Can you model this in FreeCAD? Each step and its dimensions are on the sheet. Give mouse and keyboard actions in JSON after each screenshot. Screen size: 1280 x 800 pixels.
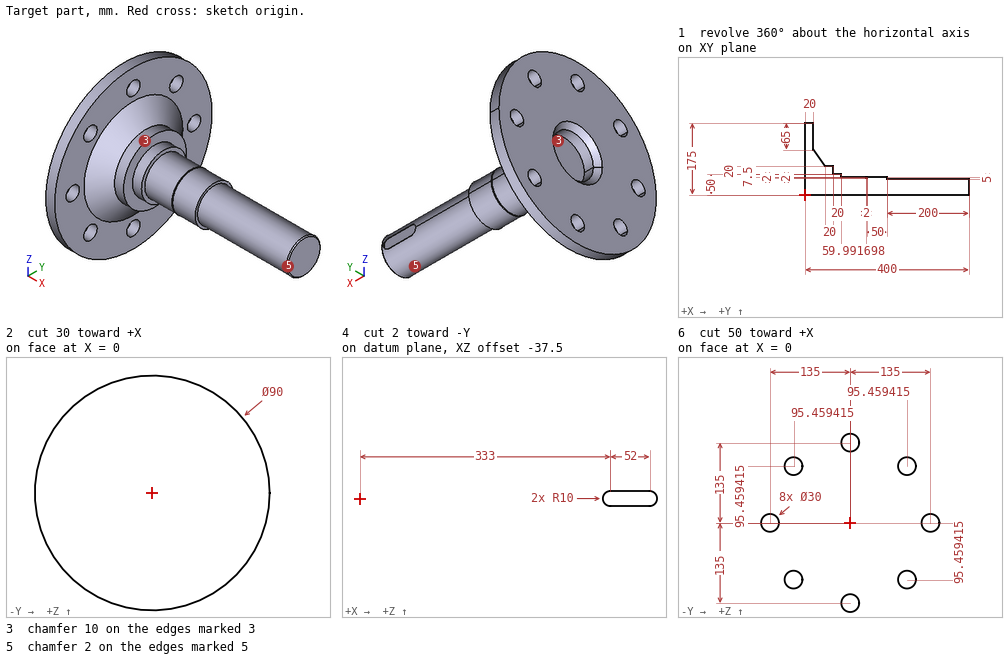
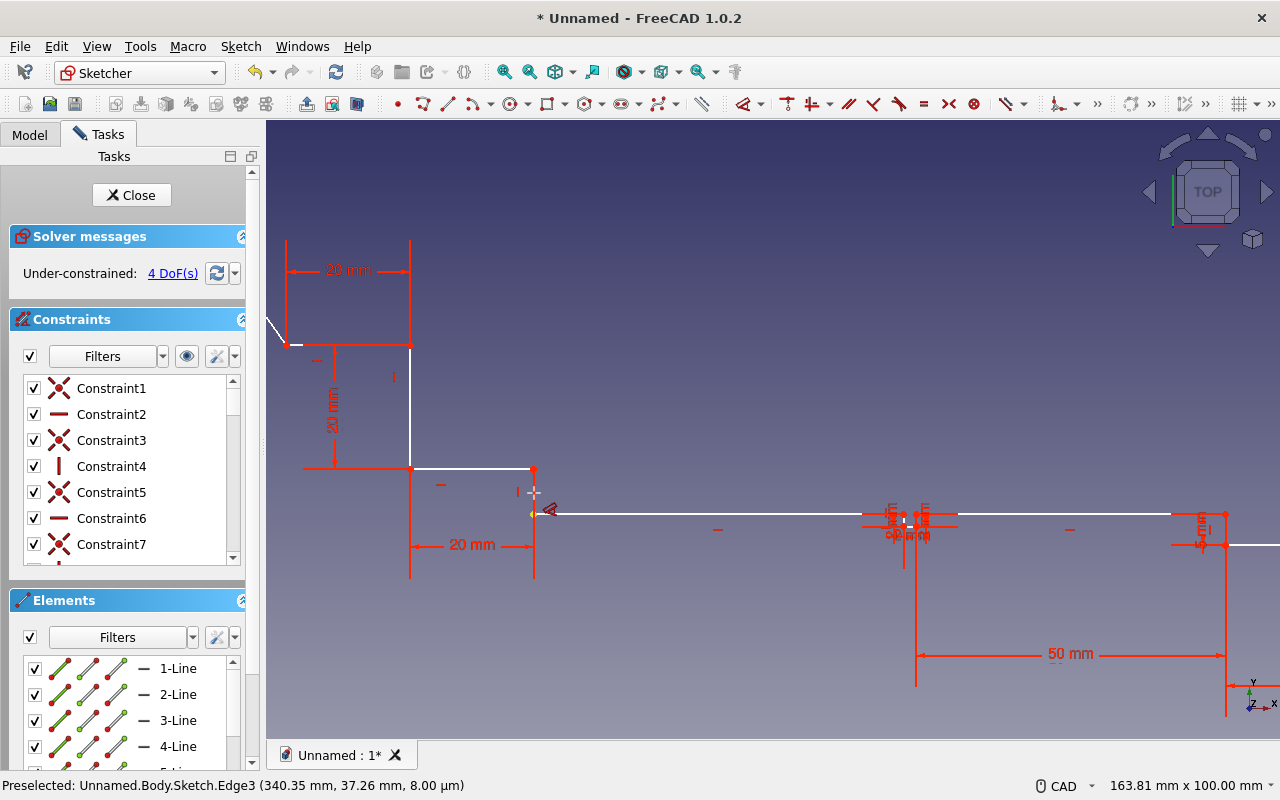
{"action": "left_click", "coordinate": [534, 492]}
{"action": "left_click", "coordinate": [500, 492]}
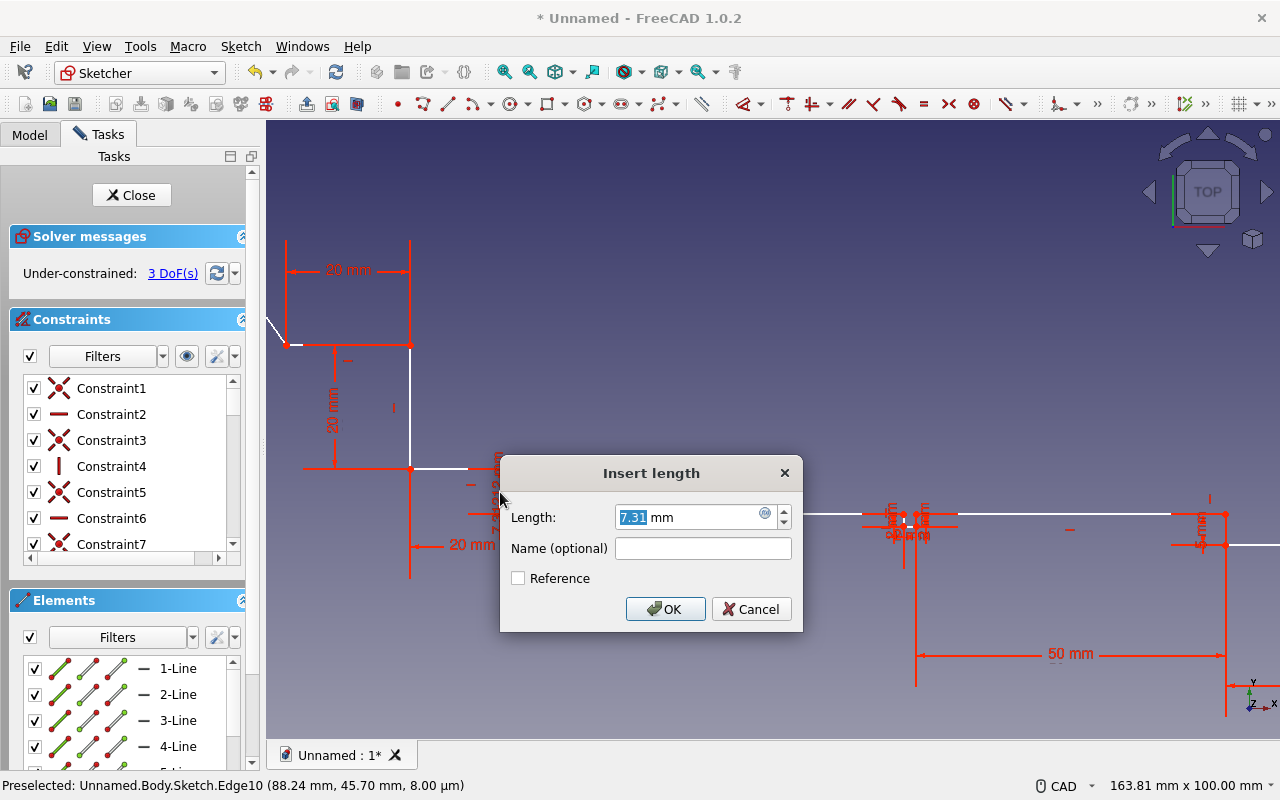
{"action": "type", "text": "7.5"}
{"action": "key", "text": "Return"}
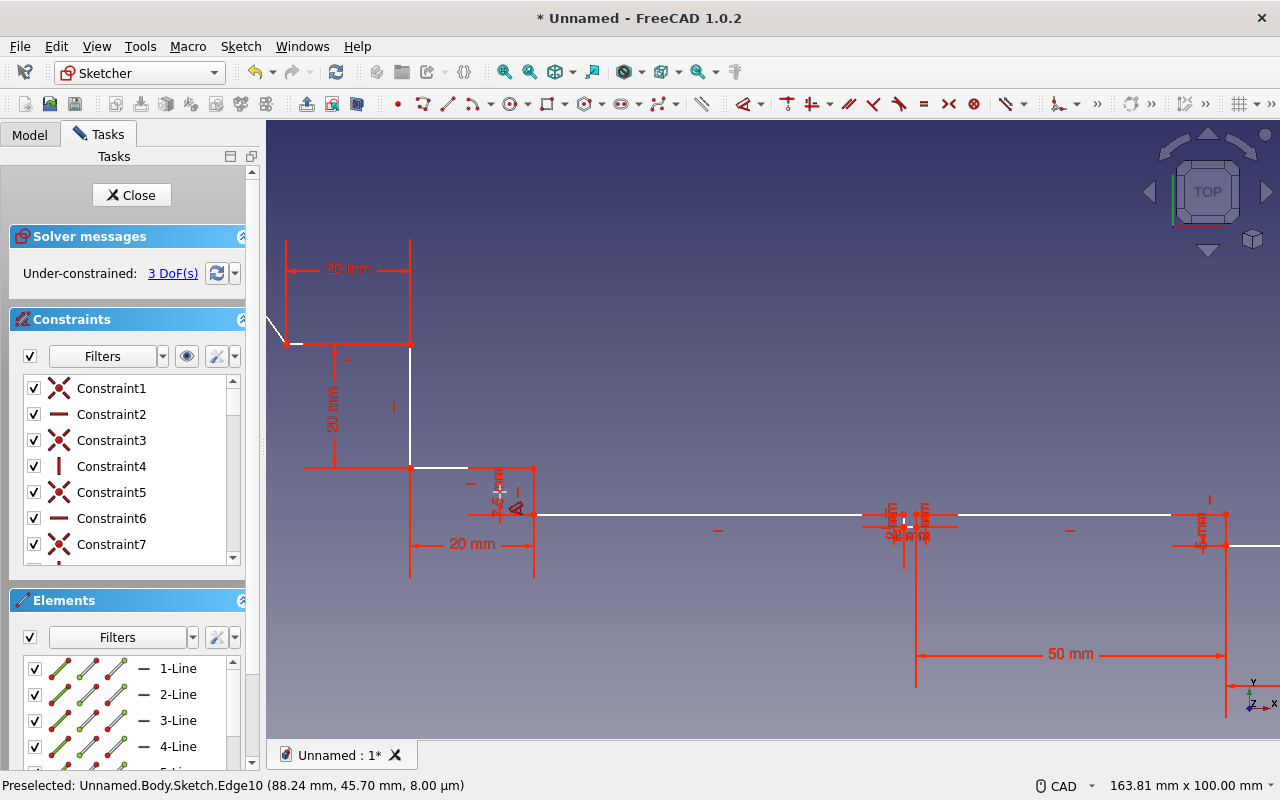
{"action": "scroll", "coordinate": [534, 493], "scroll_direction": "down", "scroll_amount": 7}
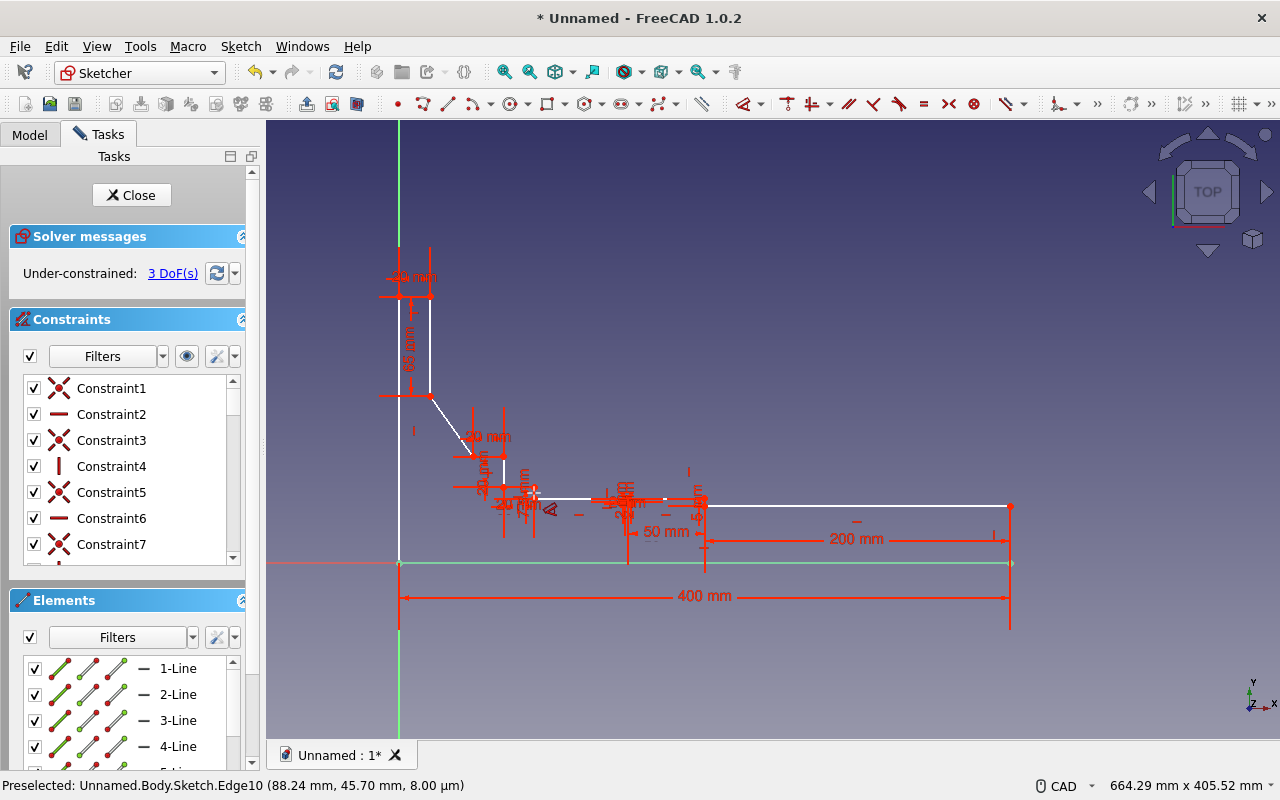
{"action": "left_click", "coordinate": [399, 377]}
{"action": "left_click", "coordinate": [365, 430]}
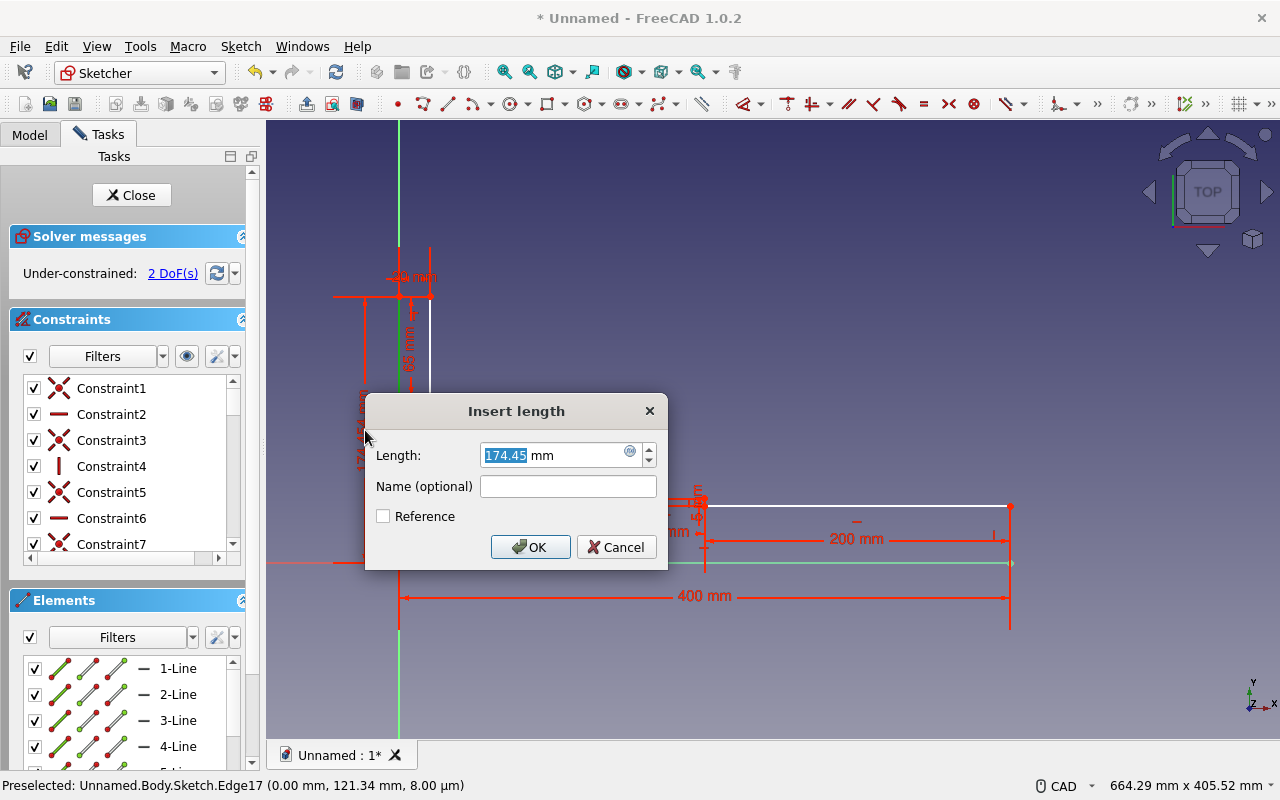
{"action": "type", "text": "175"}
{"action": "key", "text": "Return"}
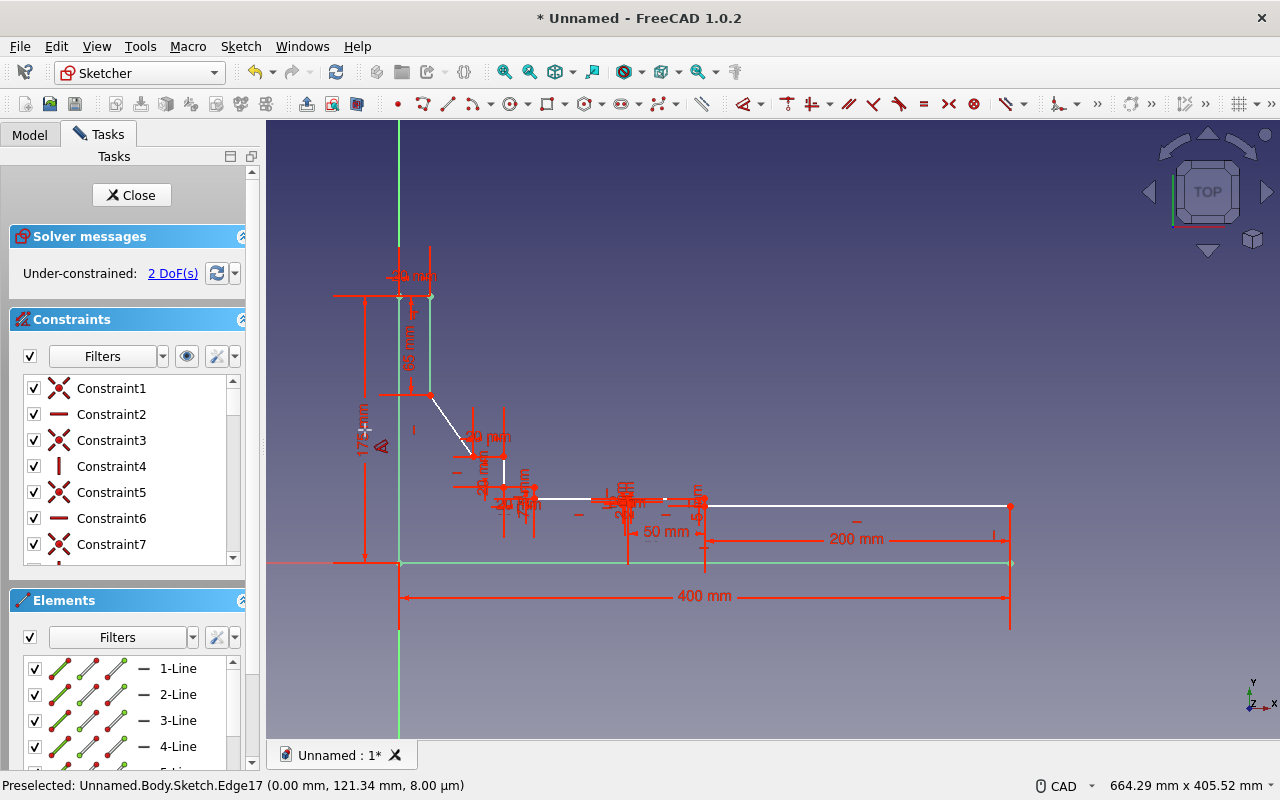
{"action": "left_click", "coordinate": [534, 487]}
{"action": "left_click", "coordinate": [365, 525]}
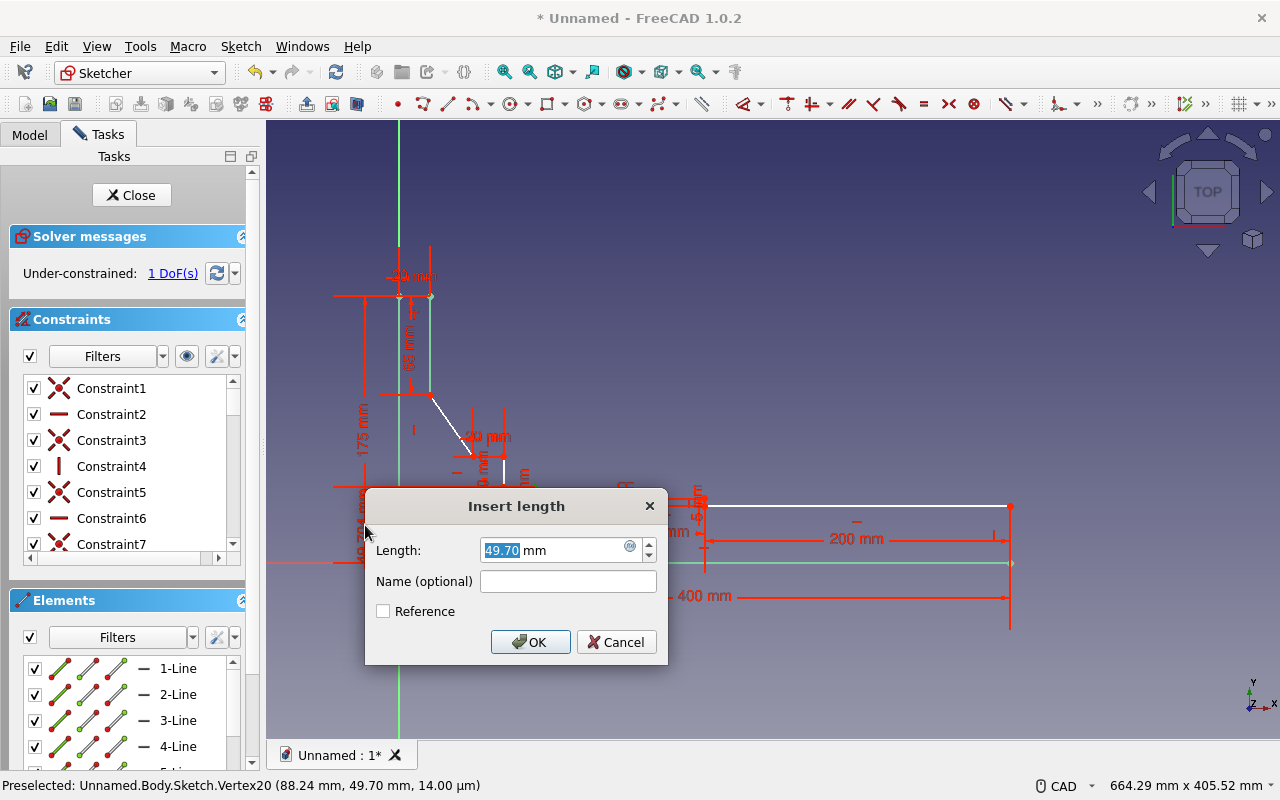
{"action": "type", "text": "50"}
{"action": "key", "text": "Return"}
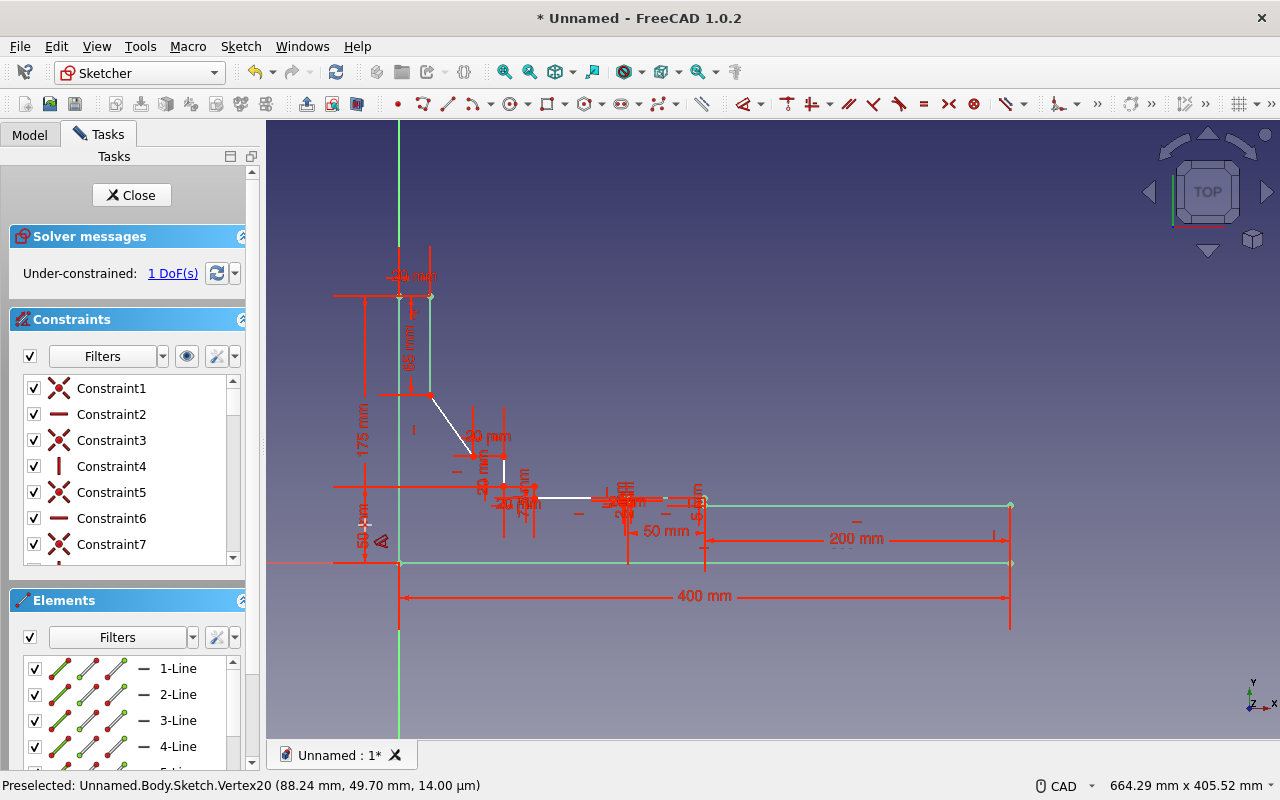
{"action": "left_click", "coordinate": [598, 498]}
{"action": "left_click", "coordinate": [580, 532]}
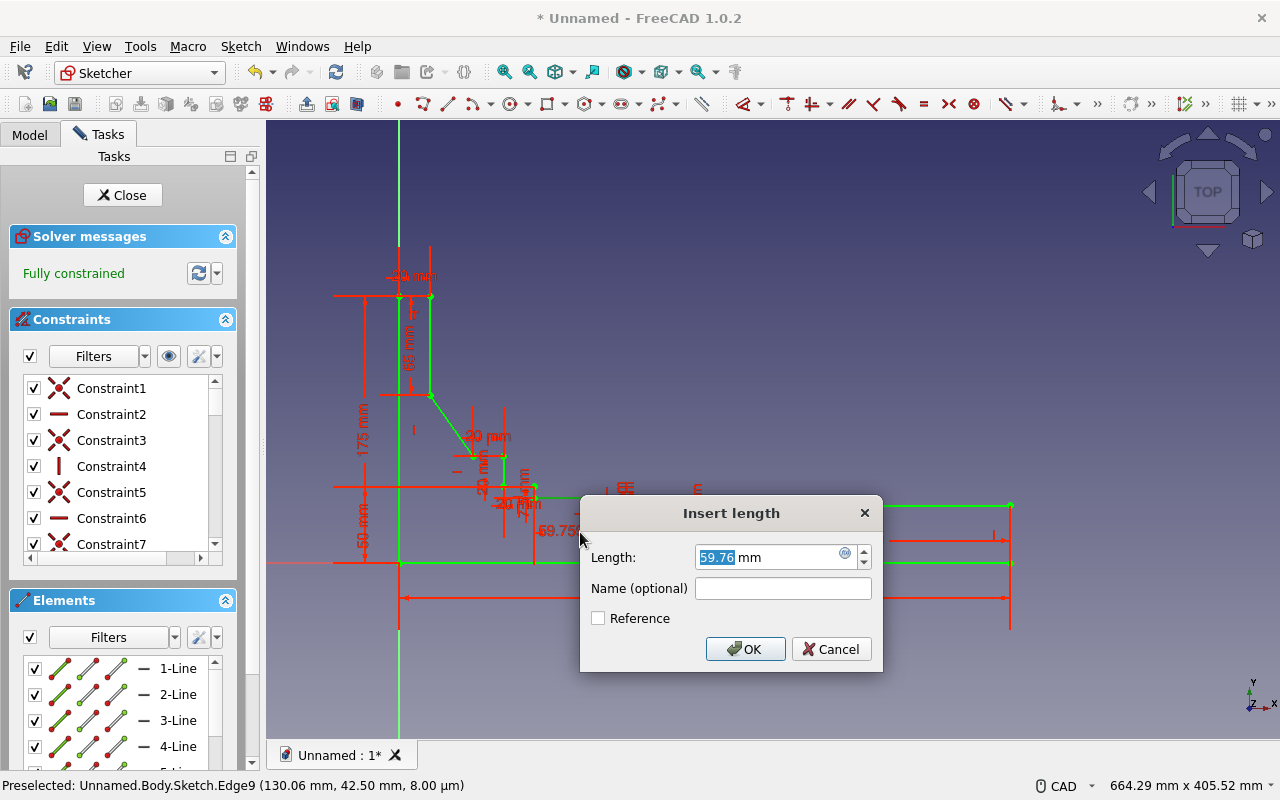
{"action": "type", "text": "59.991698"}
{"action": "key", "text": "Return"}
{"action": "key", "text": "Escape"}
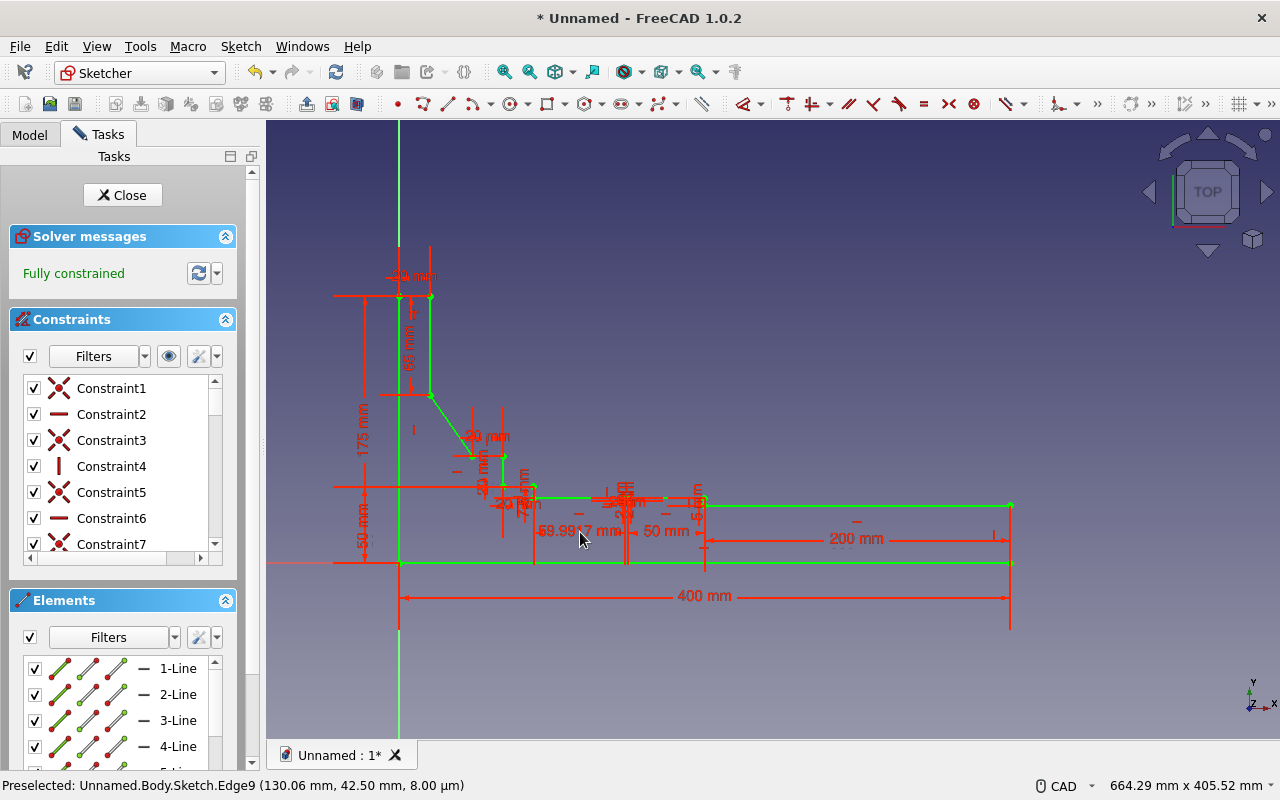
{"action": "left_click", "coordinate": [123, 195]}